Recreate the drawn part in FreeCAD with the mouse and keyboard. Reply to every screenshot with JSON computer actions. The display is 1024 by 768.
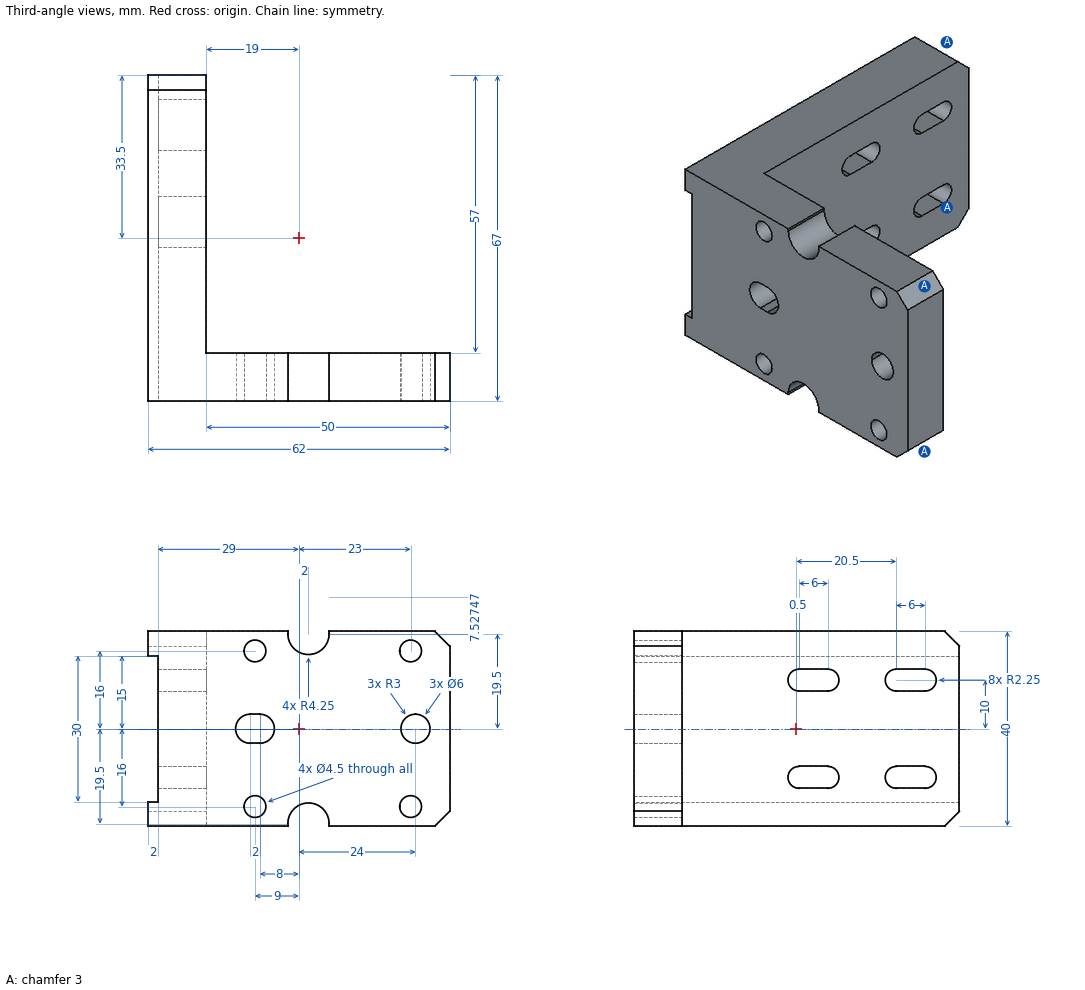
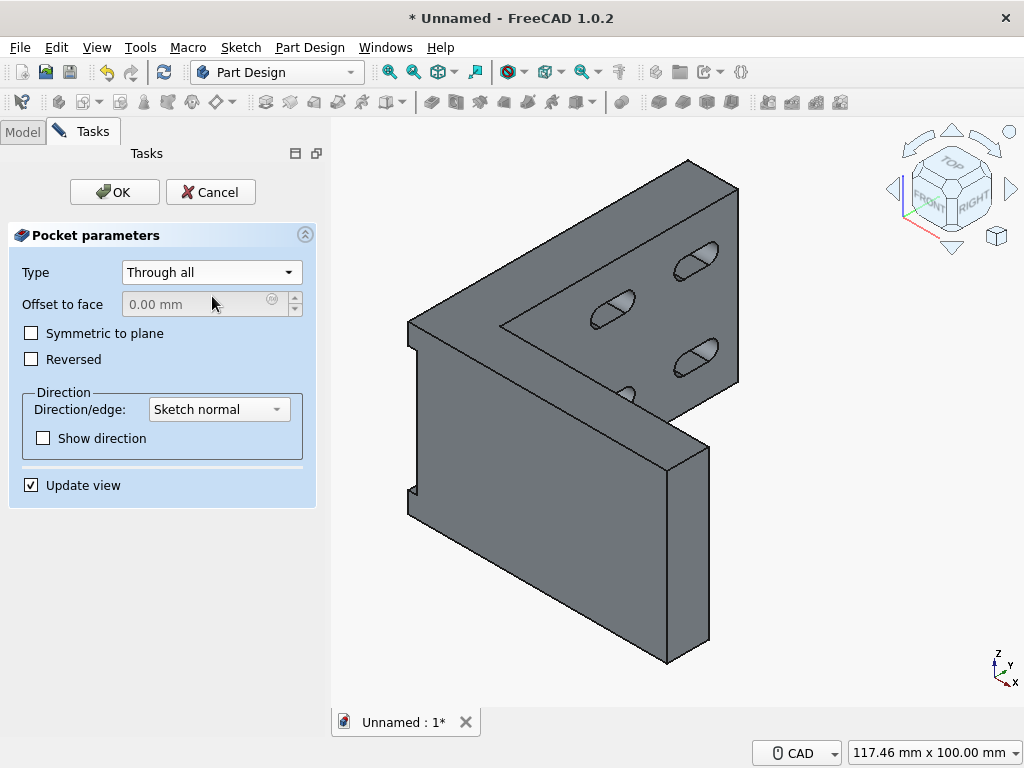
{"action": "left_click", "coordinate": [115, 192]}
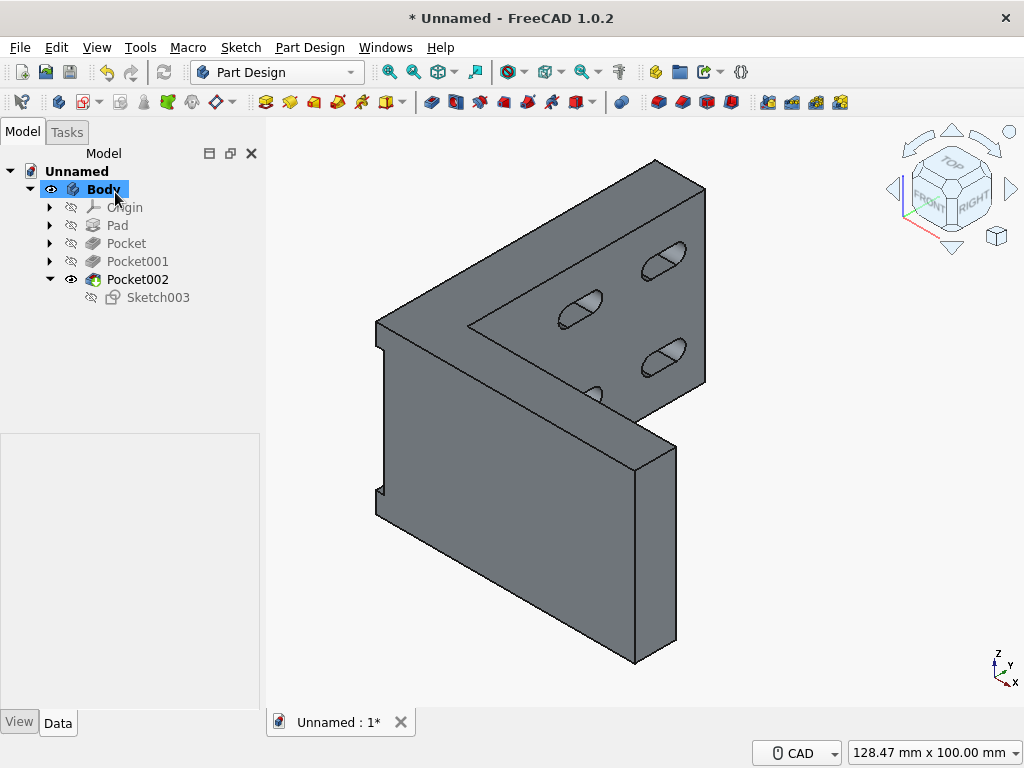
{"action": "key", "text": "4"}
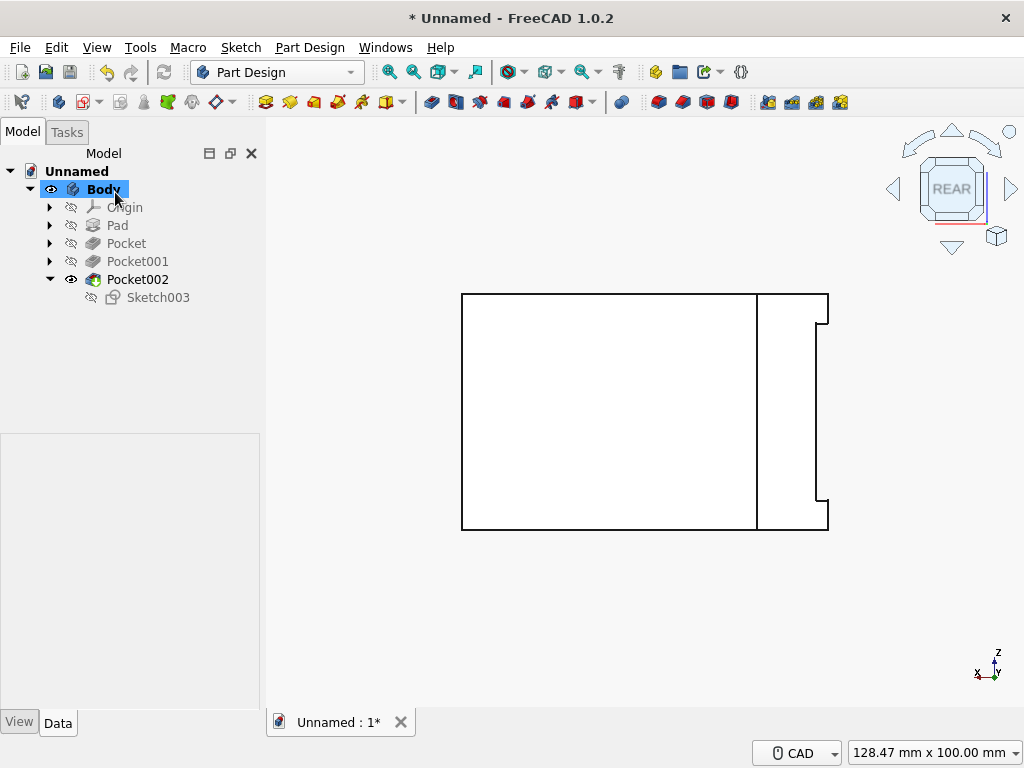
{"action": "left_click", "coordinate": [610, 411]}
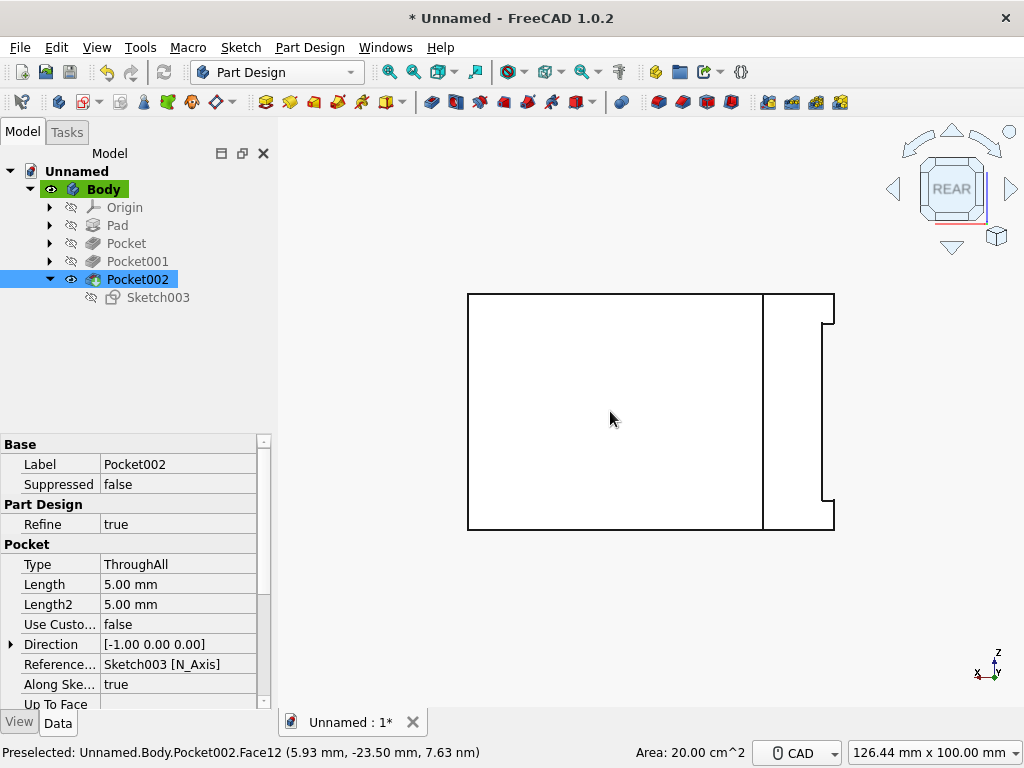
{"action": "left_click", "coordinate": [84, 102]}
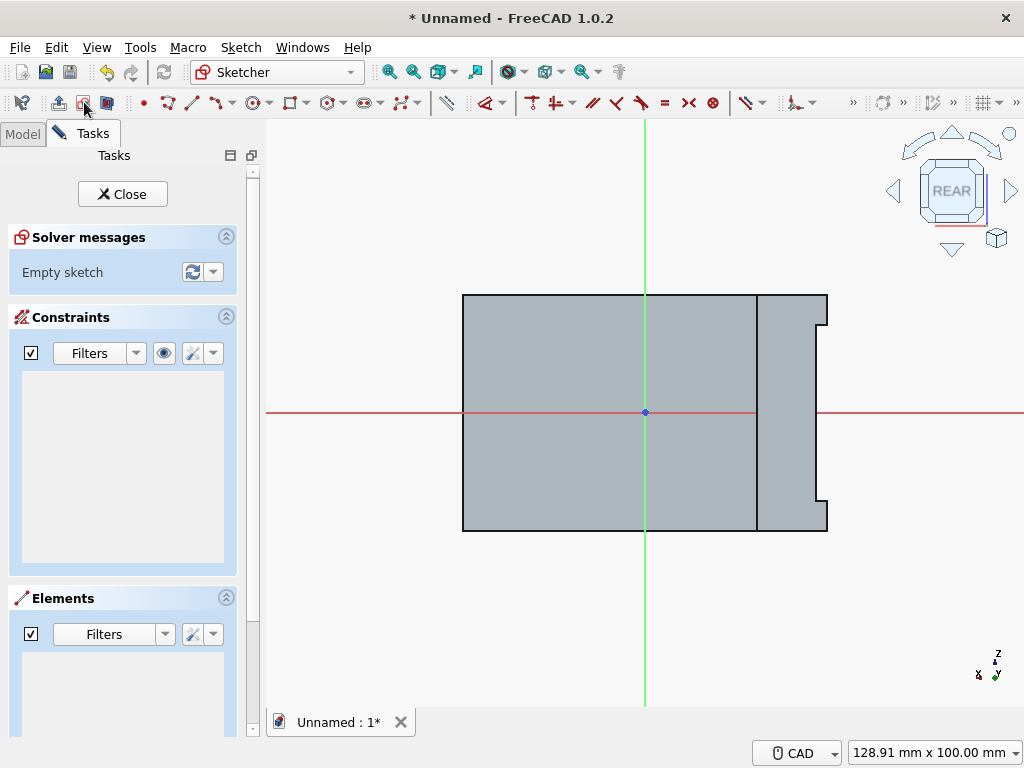
{"action": "left_click", "coordinate": [108, 104]}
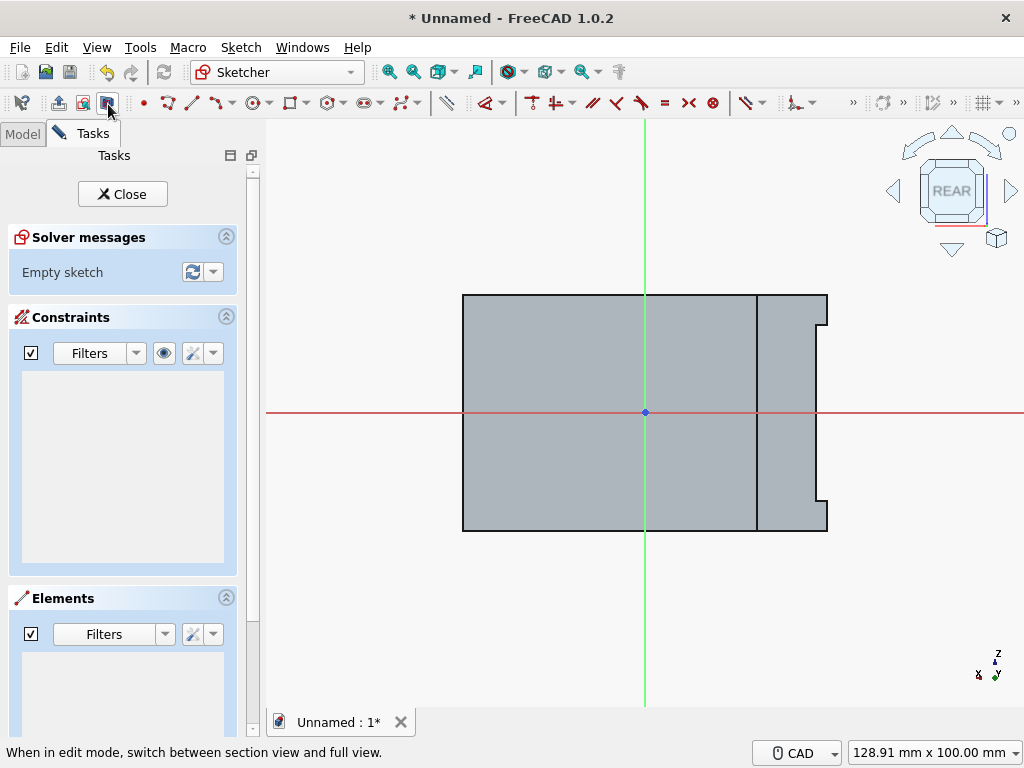
{"action": "scroll", "coordinate": [637, 413], "scroll_direction": "up", "scroll_amount": 3}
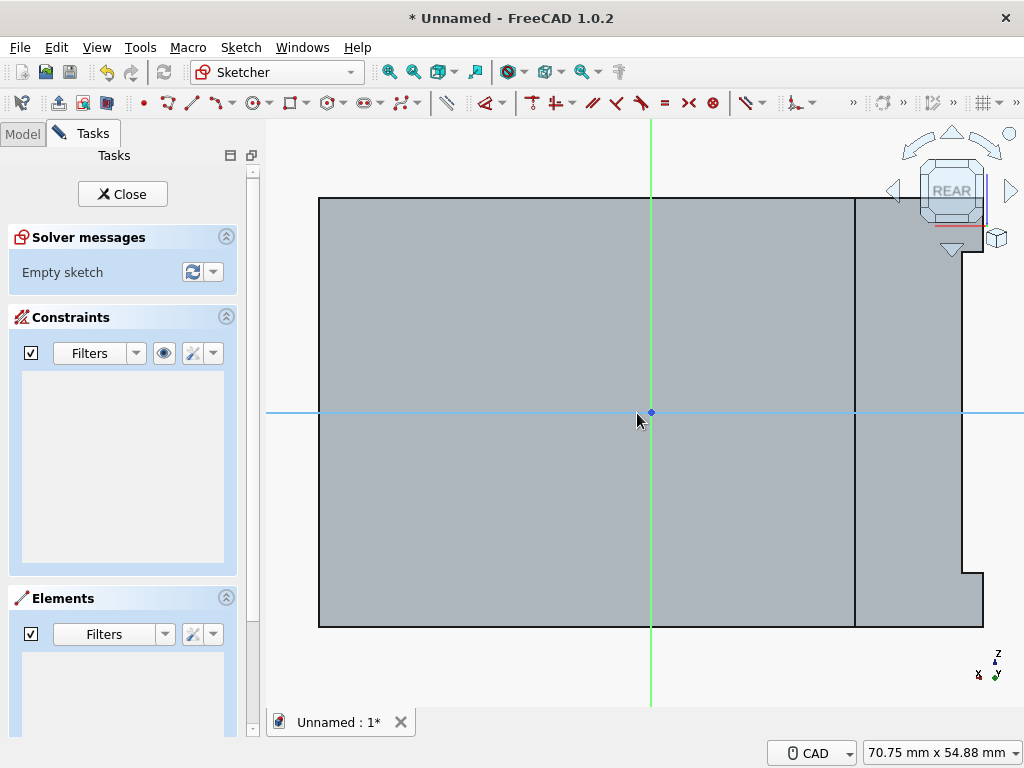
{"action": "left_click", "coordinate": [254, 104]}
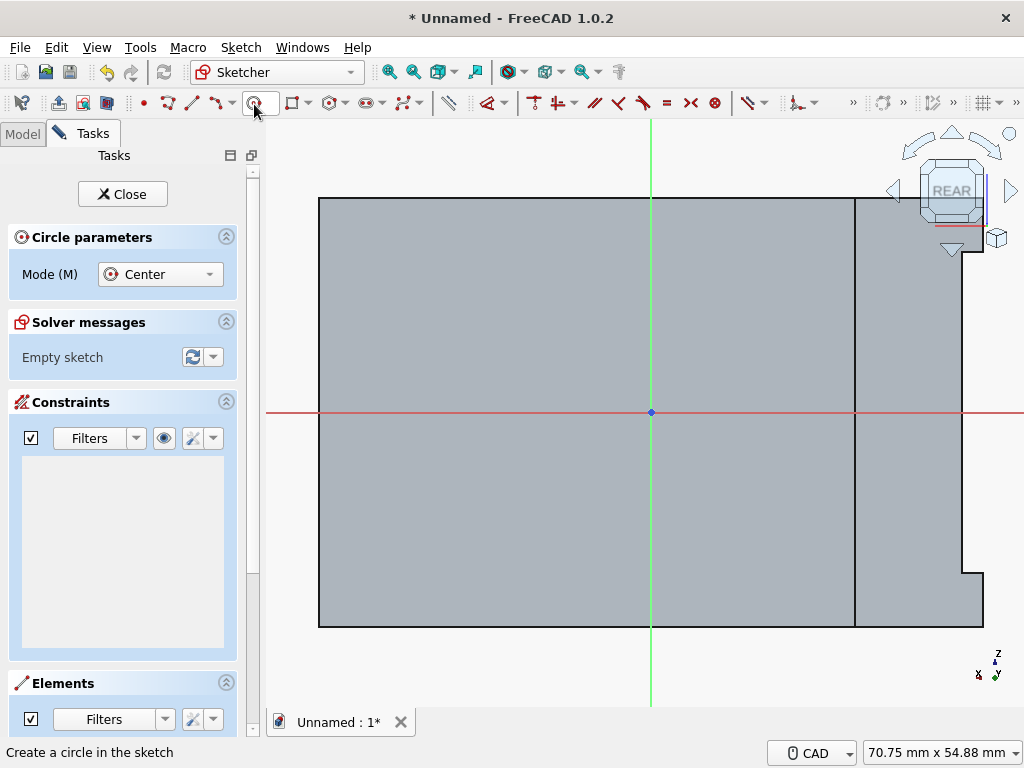
{"action": "left_click", "coordinate": [748, 584]}
{"action": "mouse_move", "coordinate": [765, 567]}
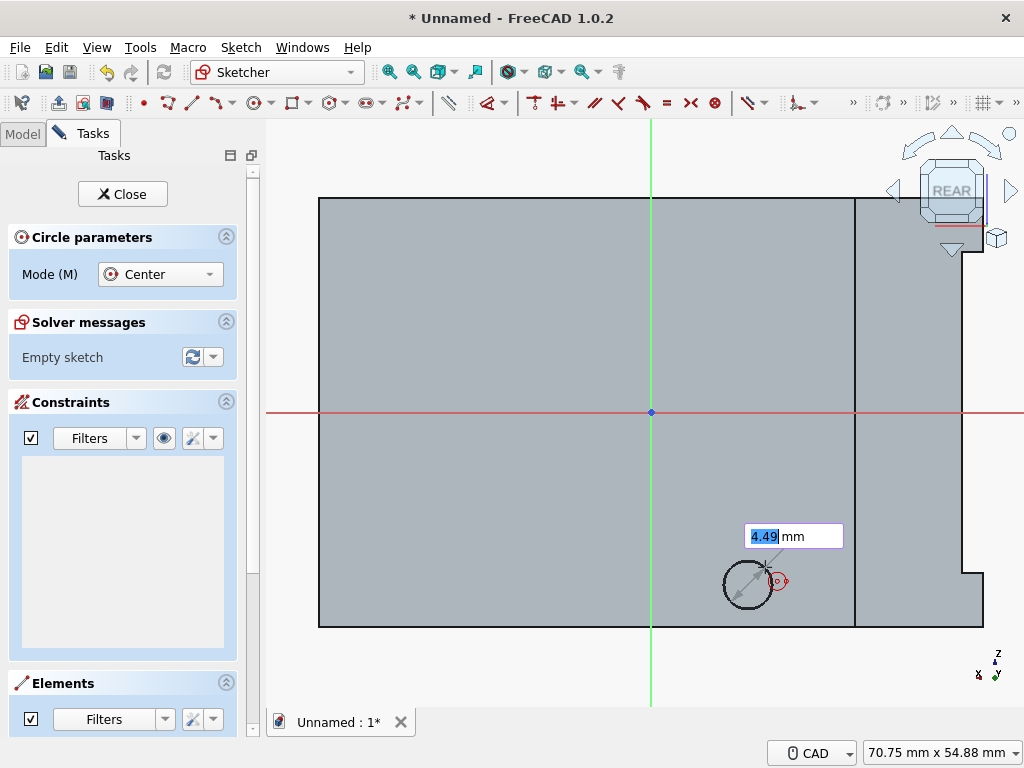
{"action": "type", "text": "4.5"}
{"action": "key", "text": "Return"}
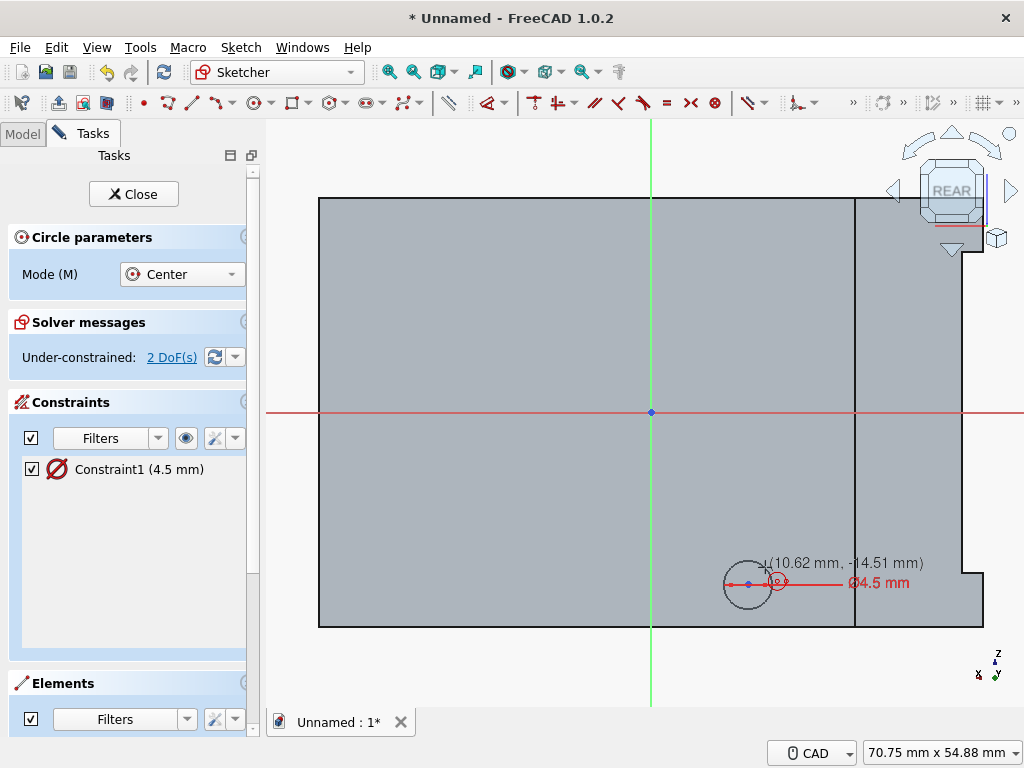
{"action": "left_click", "coordinate": [748, 241]}
{"action": "mouse_move", "coordinate": [765, 224]}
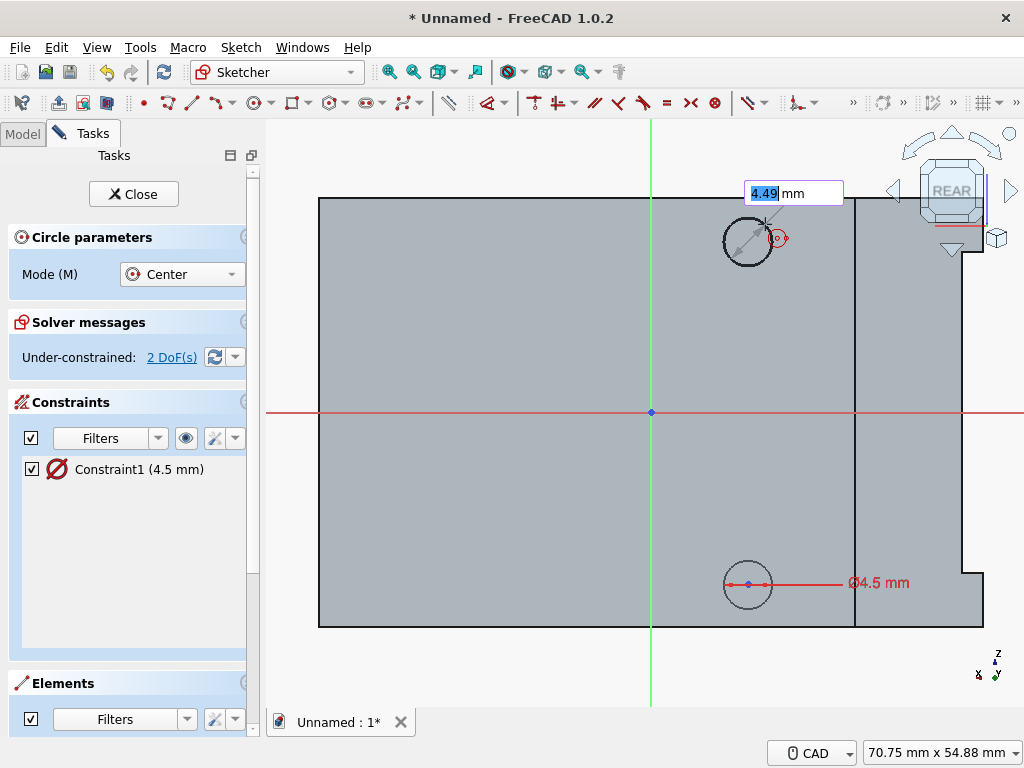
{"action": "type", "text": "4.5"}
{"action": "key", "text": "Return"}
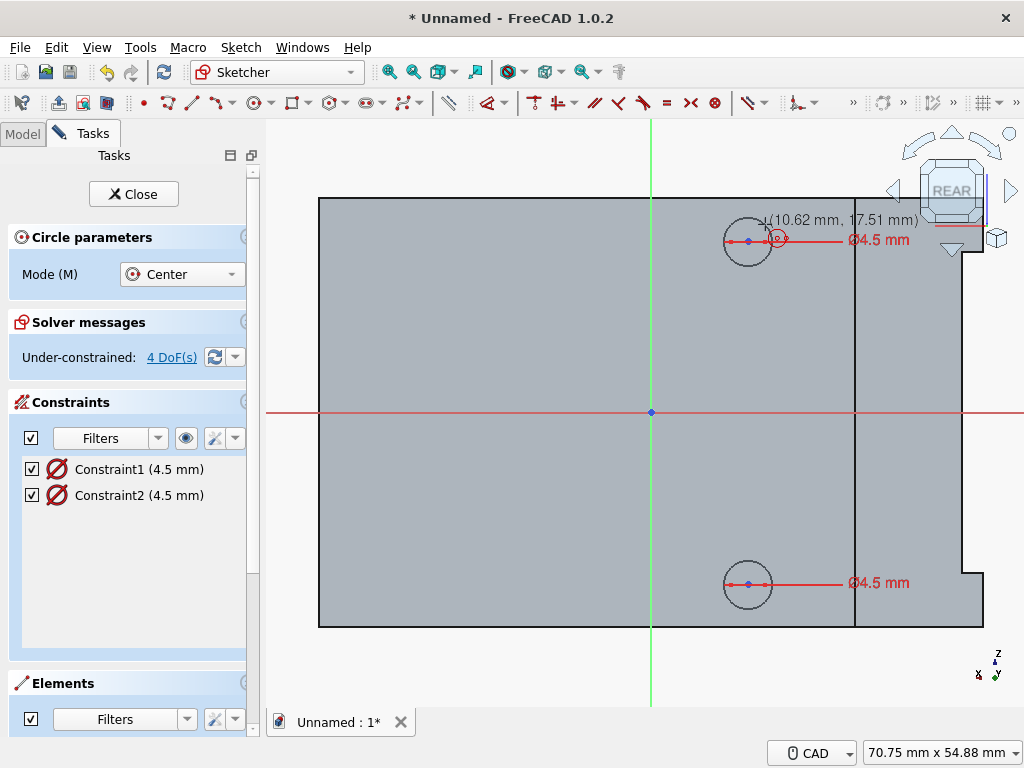
{"action": "left_click", "coordinate": [405, 241]}
{"action": "mouse_move", "coordinate": [422, 224]}